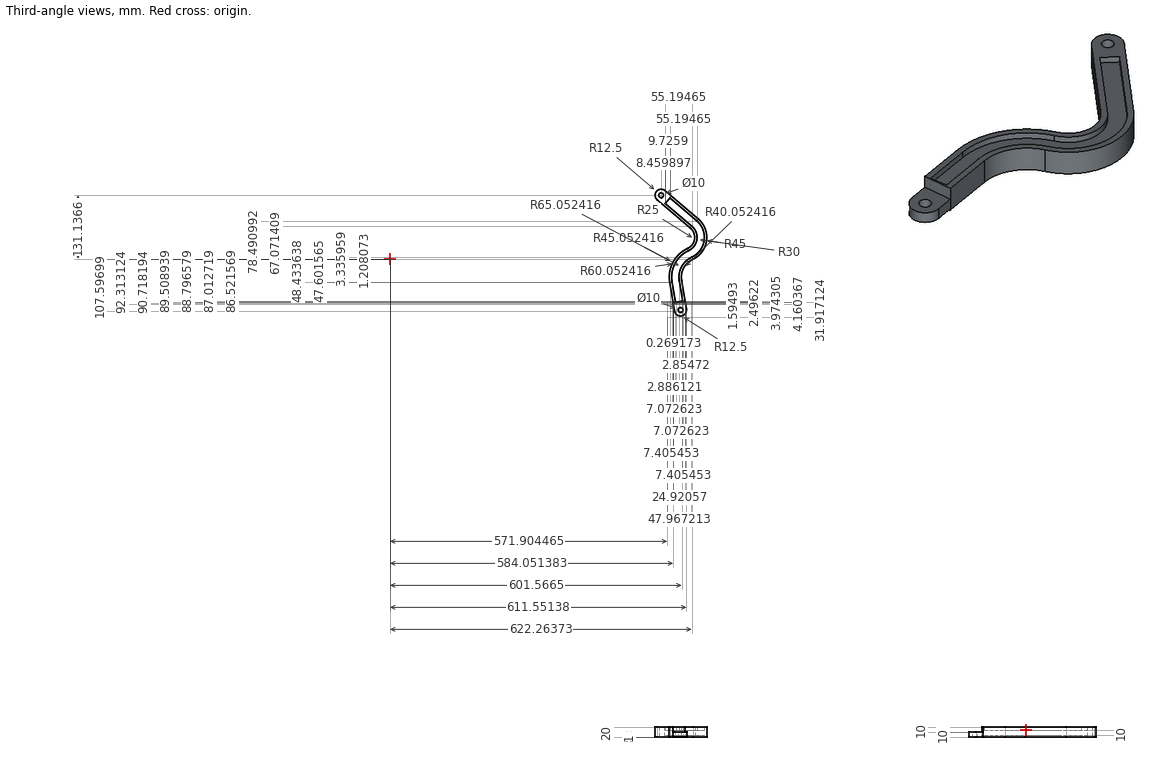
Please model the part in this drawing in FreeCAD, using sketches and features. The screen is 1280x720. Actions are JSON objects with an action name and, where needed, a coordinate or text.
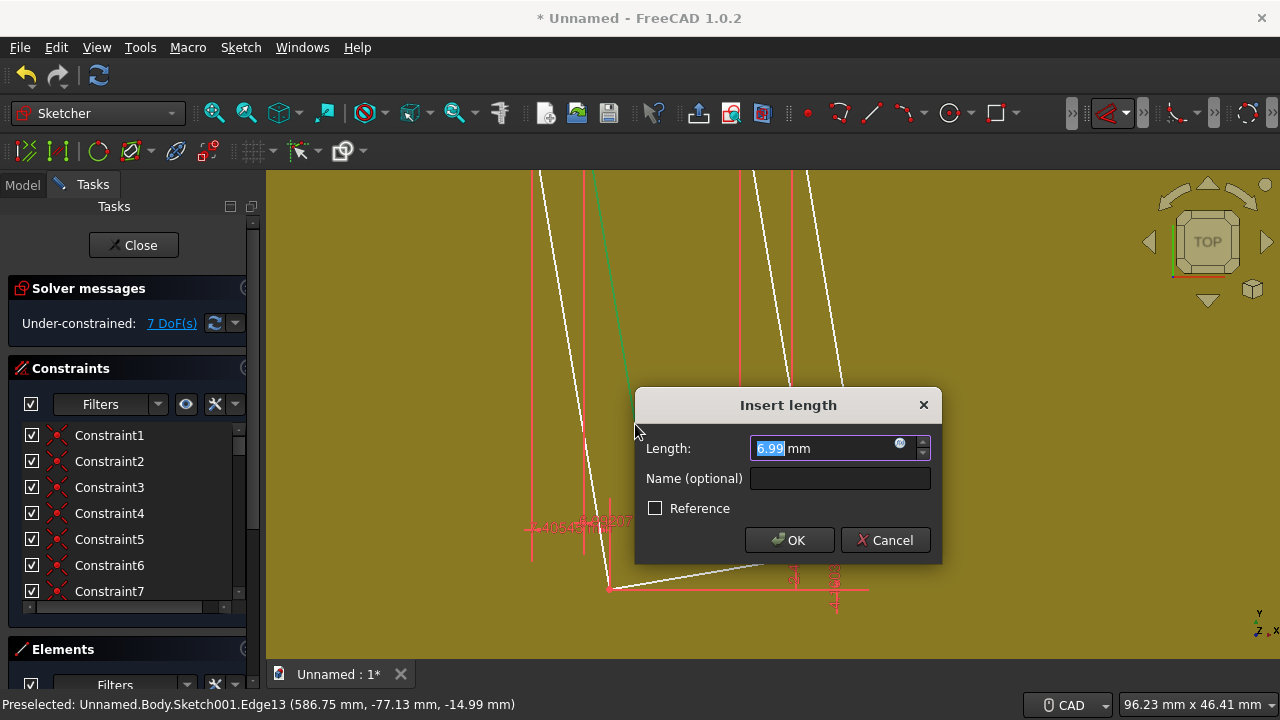
{"action": "type", "text": "7.072623"}
{"action": "key", "text": "Return"}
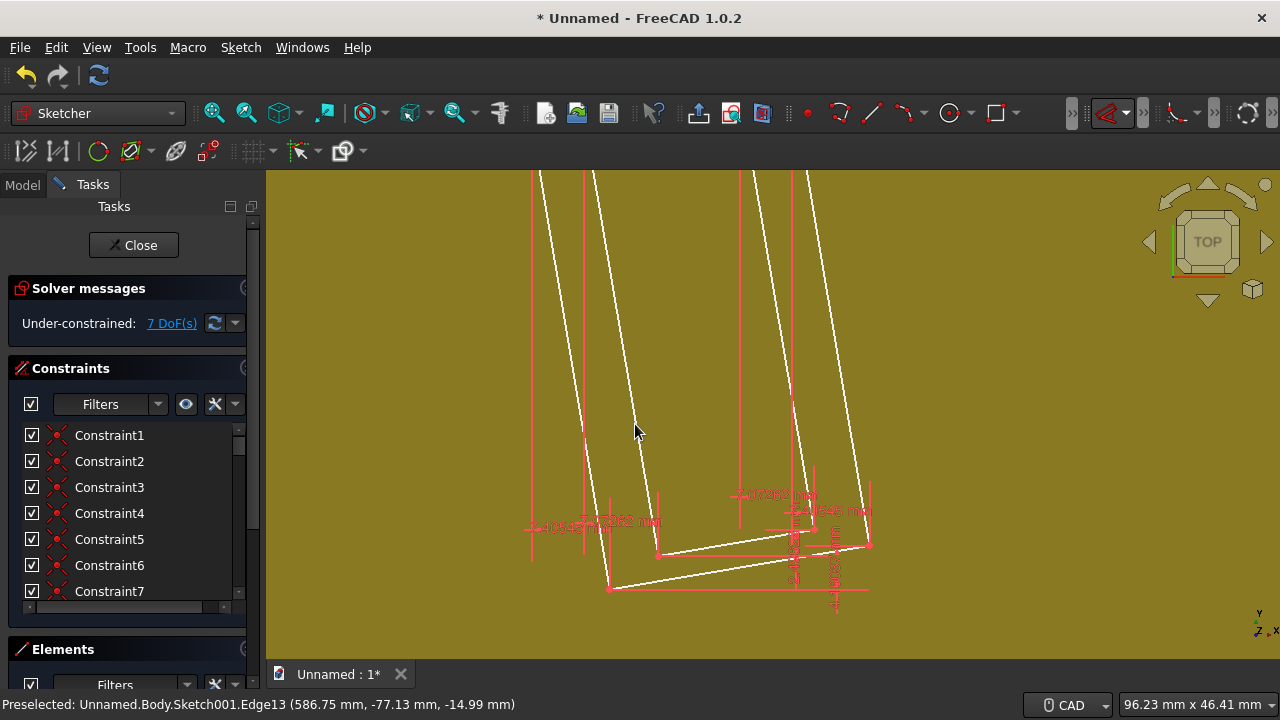
{"action": "scroll", "coordinate": [691, 580], "scroll_direction": "down", "scroll_amount": 10}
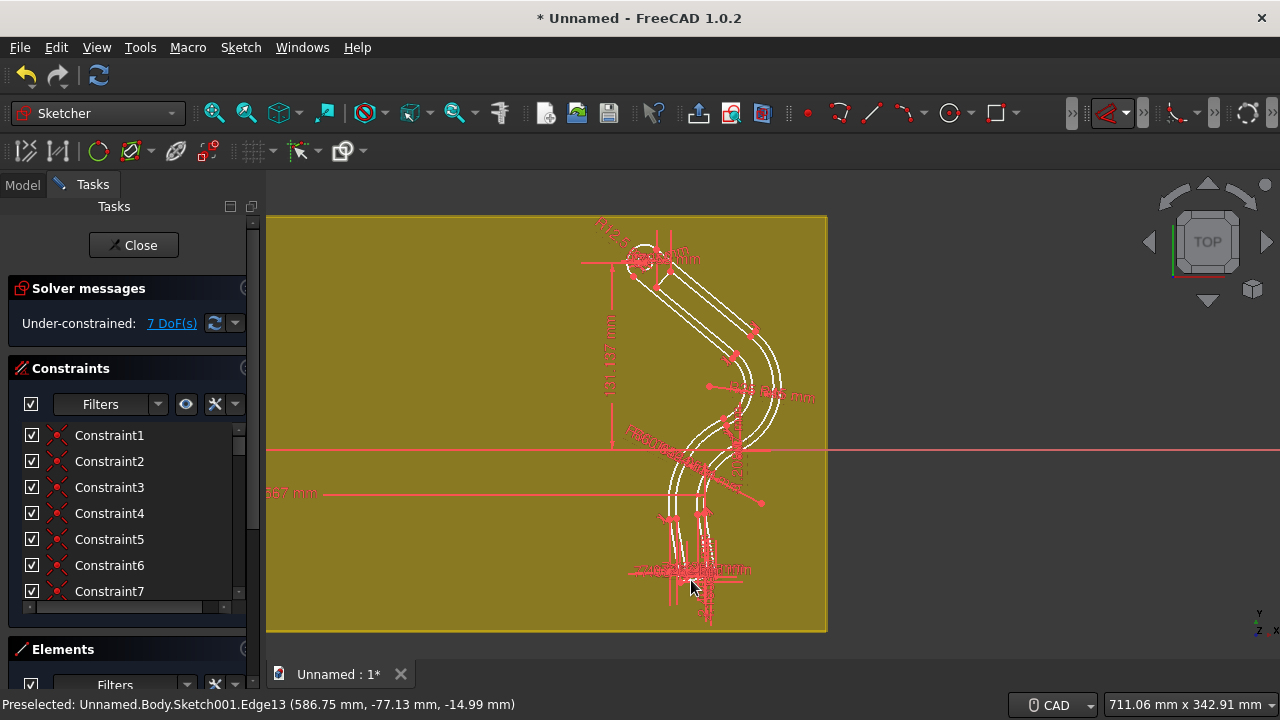
{"action": "scroll", "coordinate": [713, 333], "scroll_direction": "up", "scroll_amount": 4}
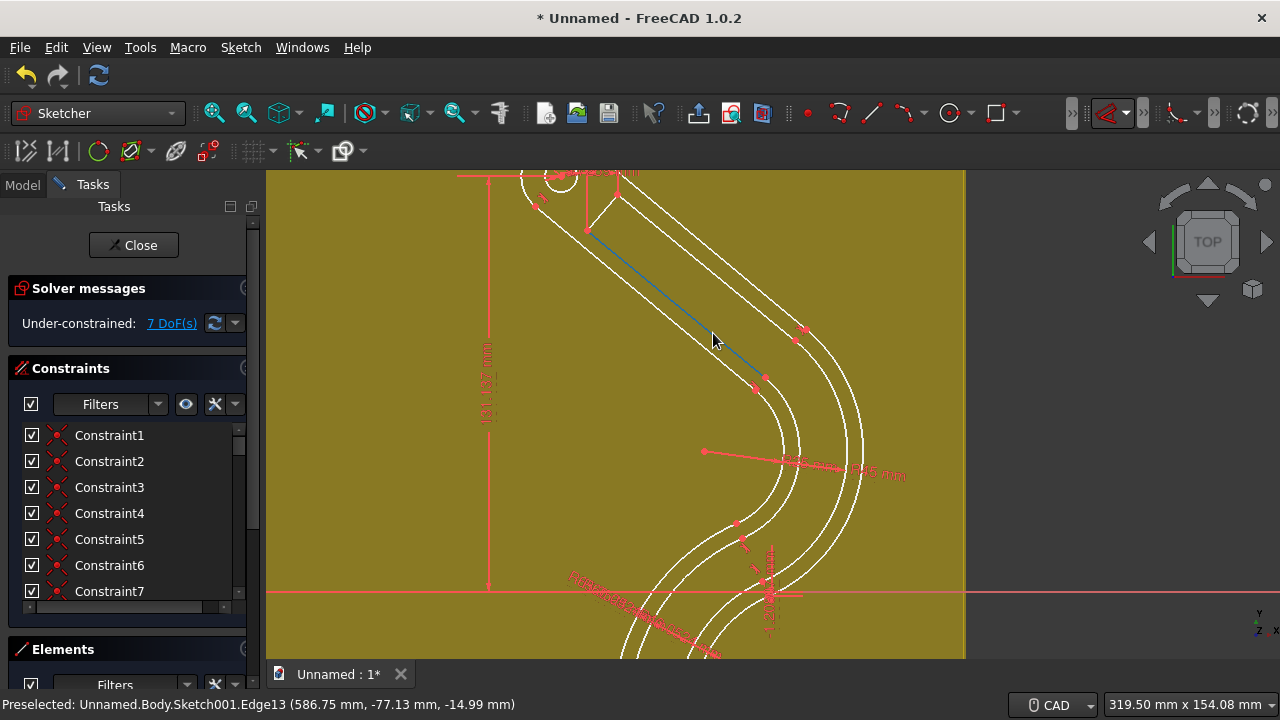
{"action": "left_click", "coordinate": [712, 334]}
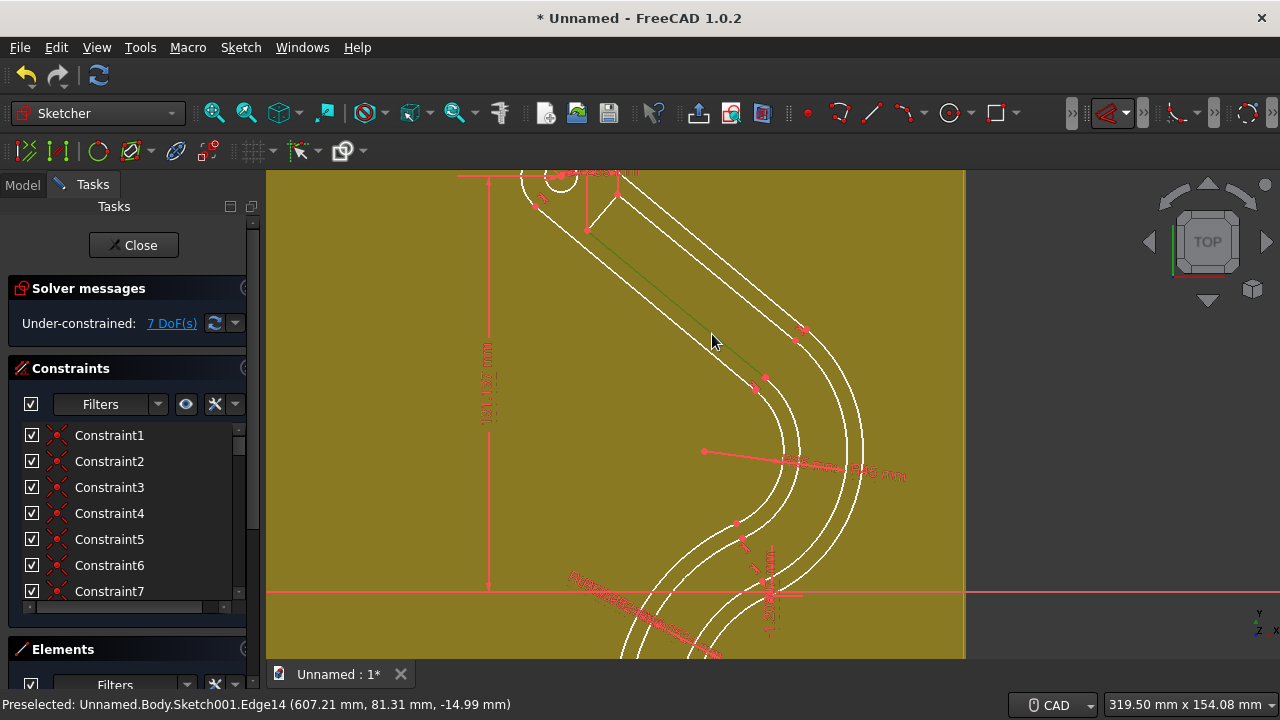
{"action": "key", "text": "l"}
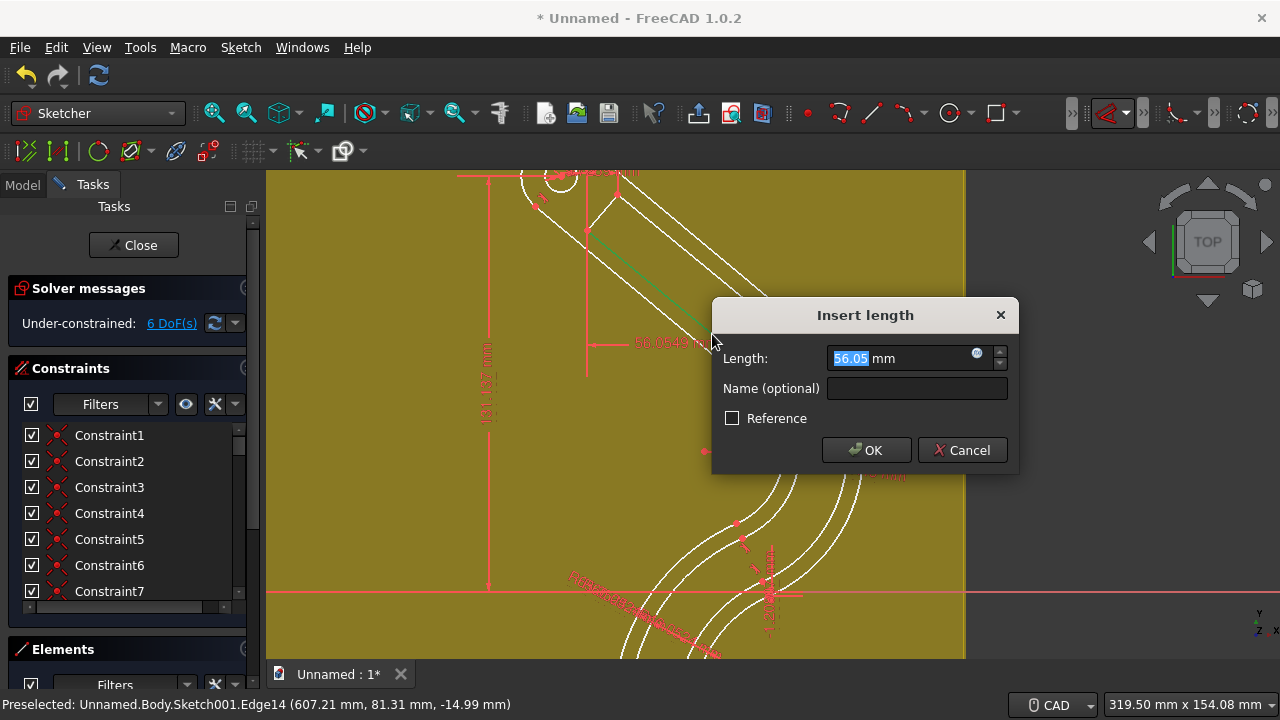
{"action": "type", "text": "55.19465"}
{"action": "key", "text": "Return"}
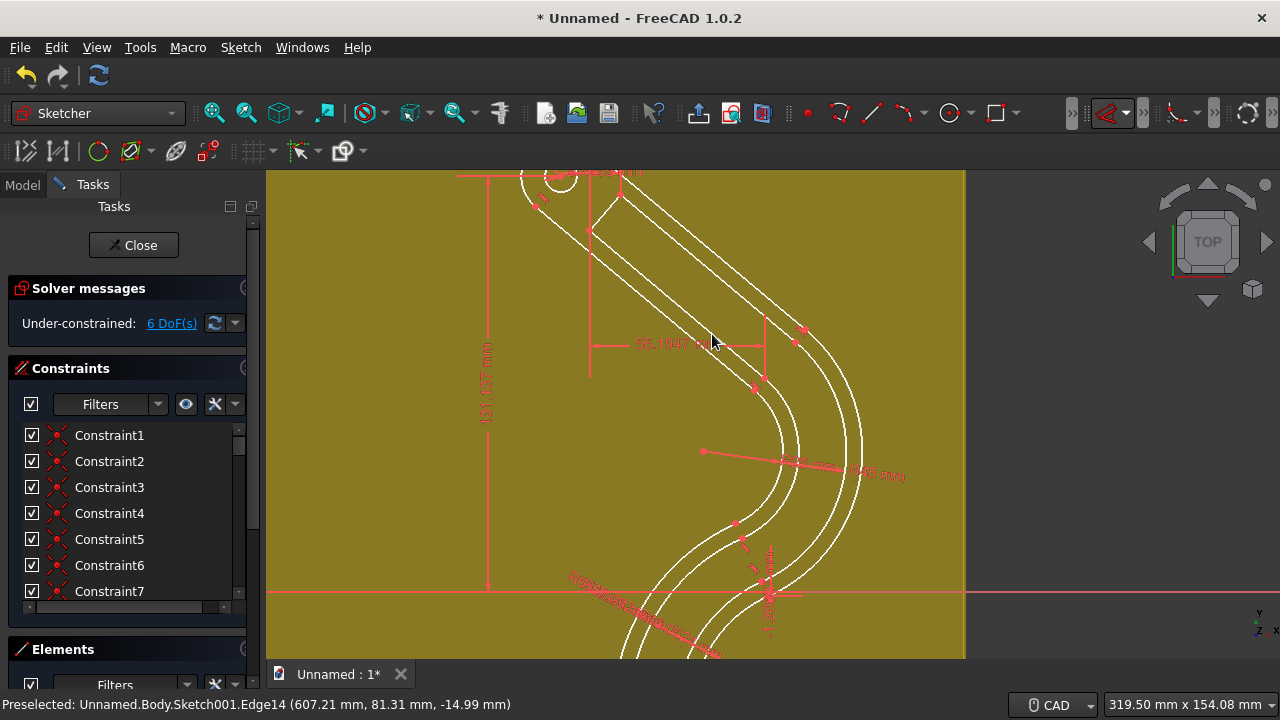
{"action": "left_click", "coordinate": [673, 239]}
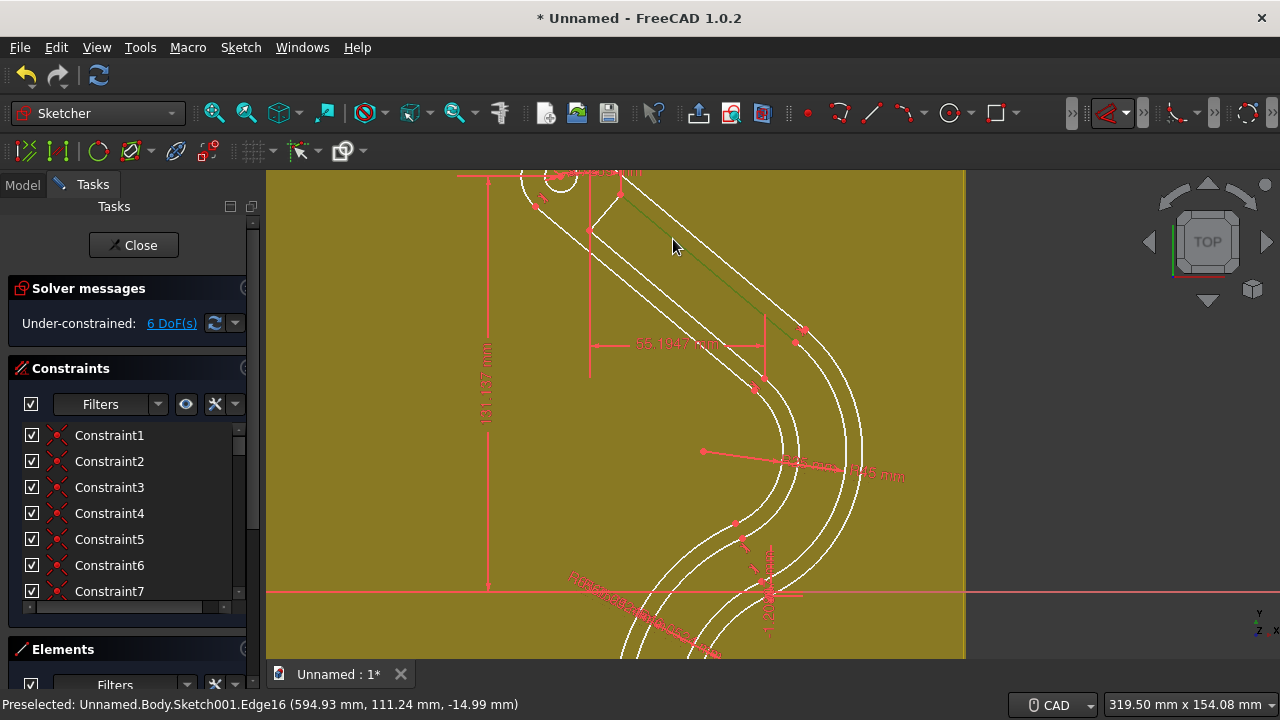
{"action": "key", "text": "l"}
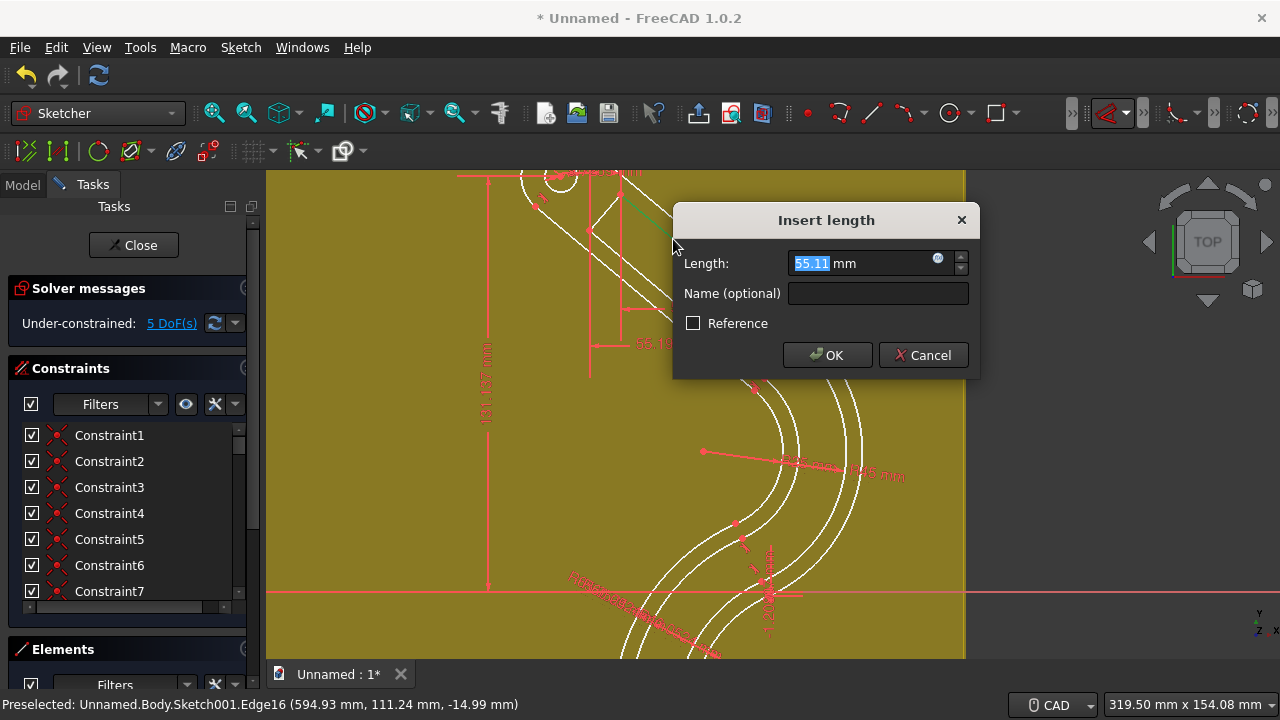
{"action": "type", "text": "55.19465"}
{"action": "key", "text": "Return"}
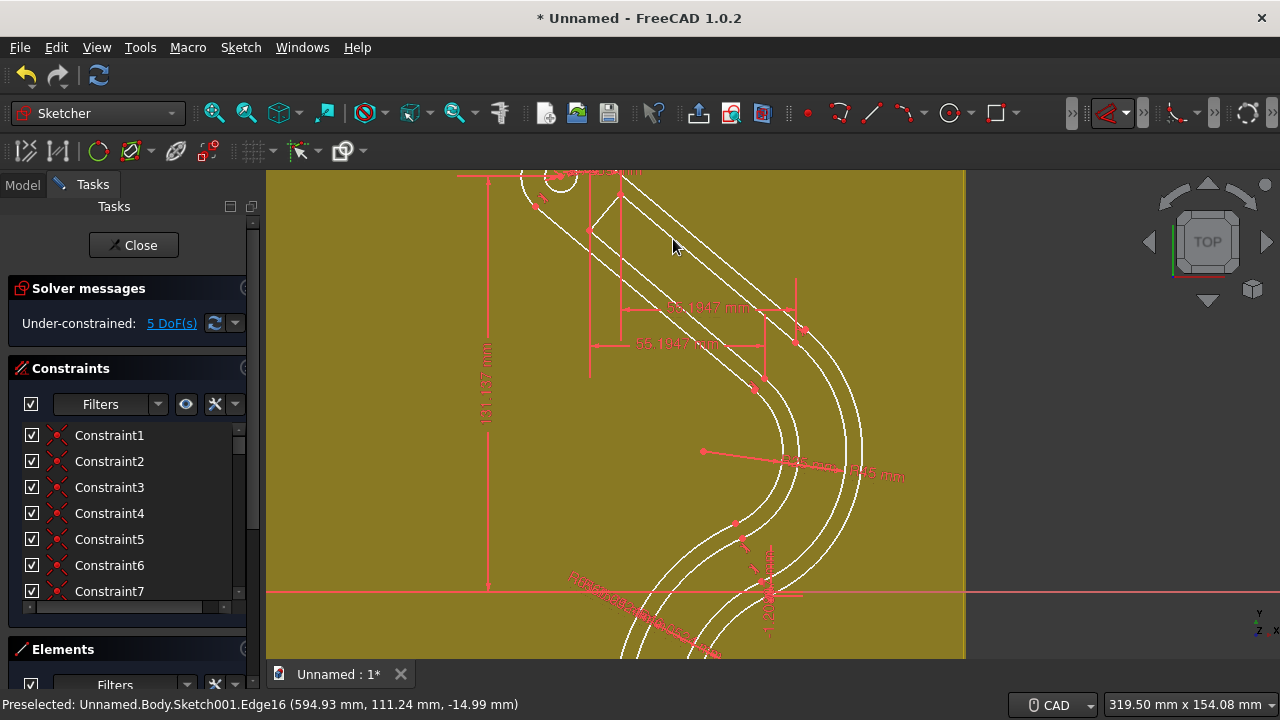
{"action": "scroll", "coordinate": [590, 231], "scroll_direction": "up", "scroll_amount": 2}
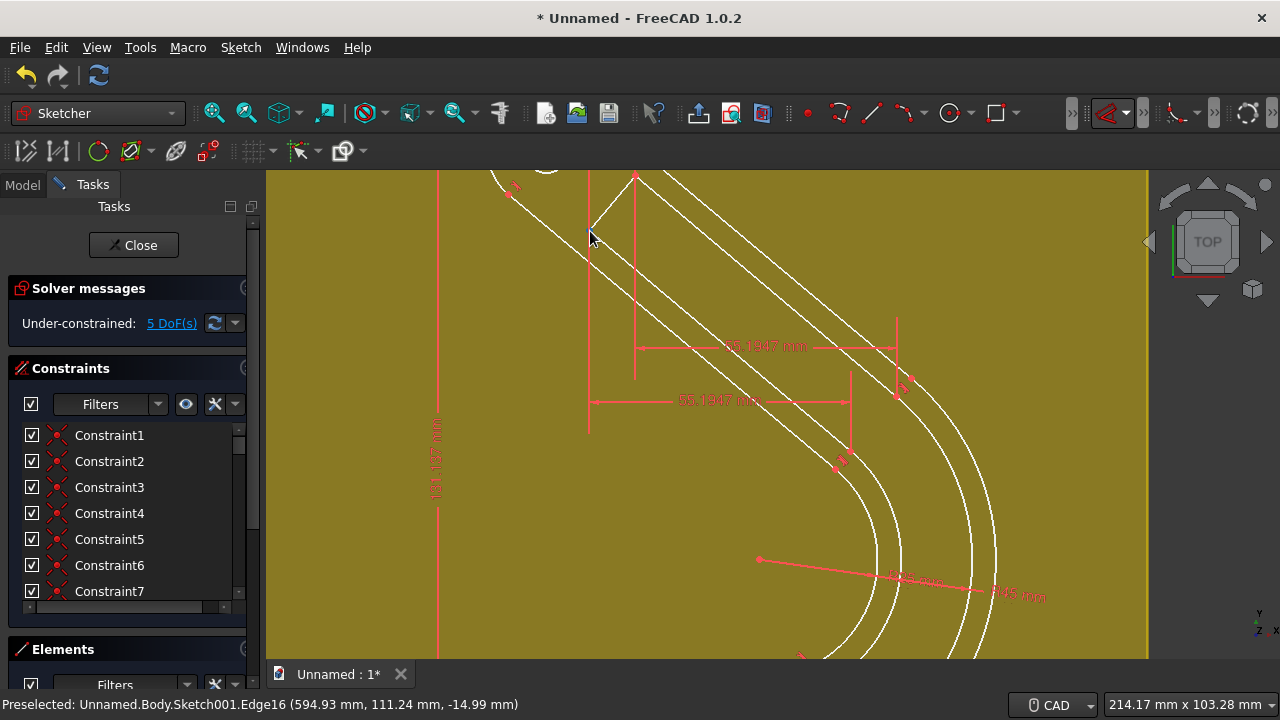
{"action": "left_click", "coordinate": [589, 231]}